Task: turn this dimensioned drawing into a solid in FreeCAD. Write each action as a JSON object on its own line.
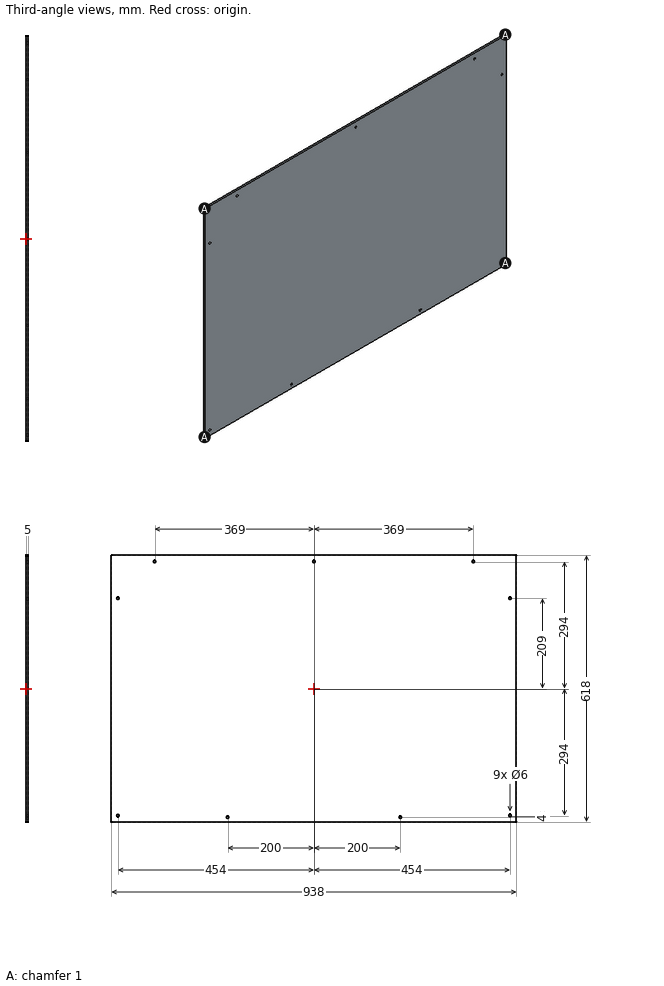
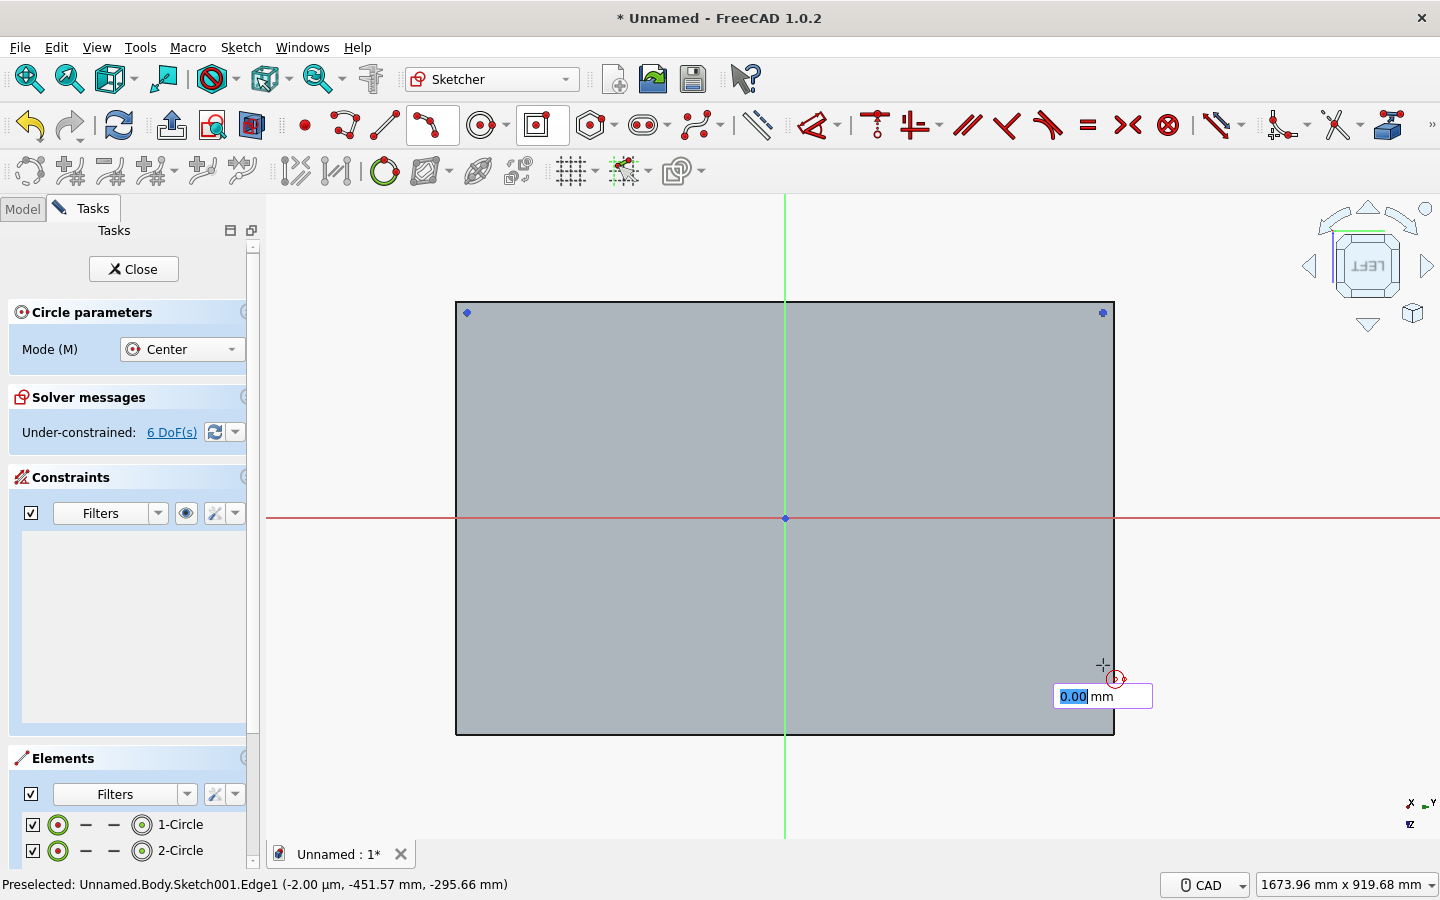
{"action": "scroll", "coordinate": [1105, 663], "scroll_direction": "up", "scroll_amount": 11}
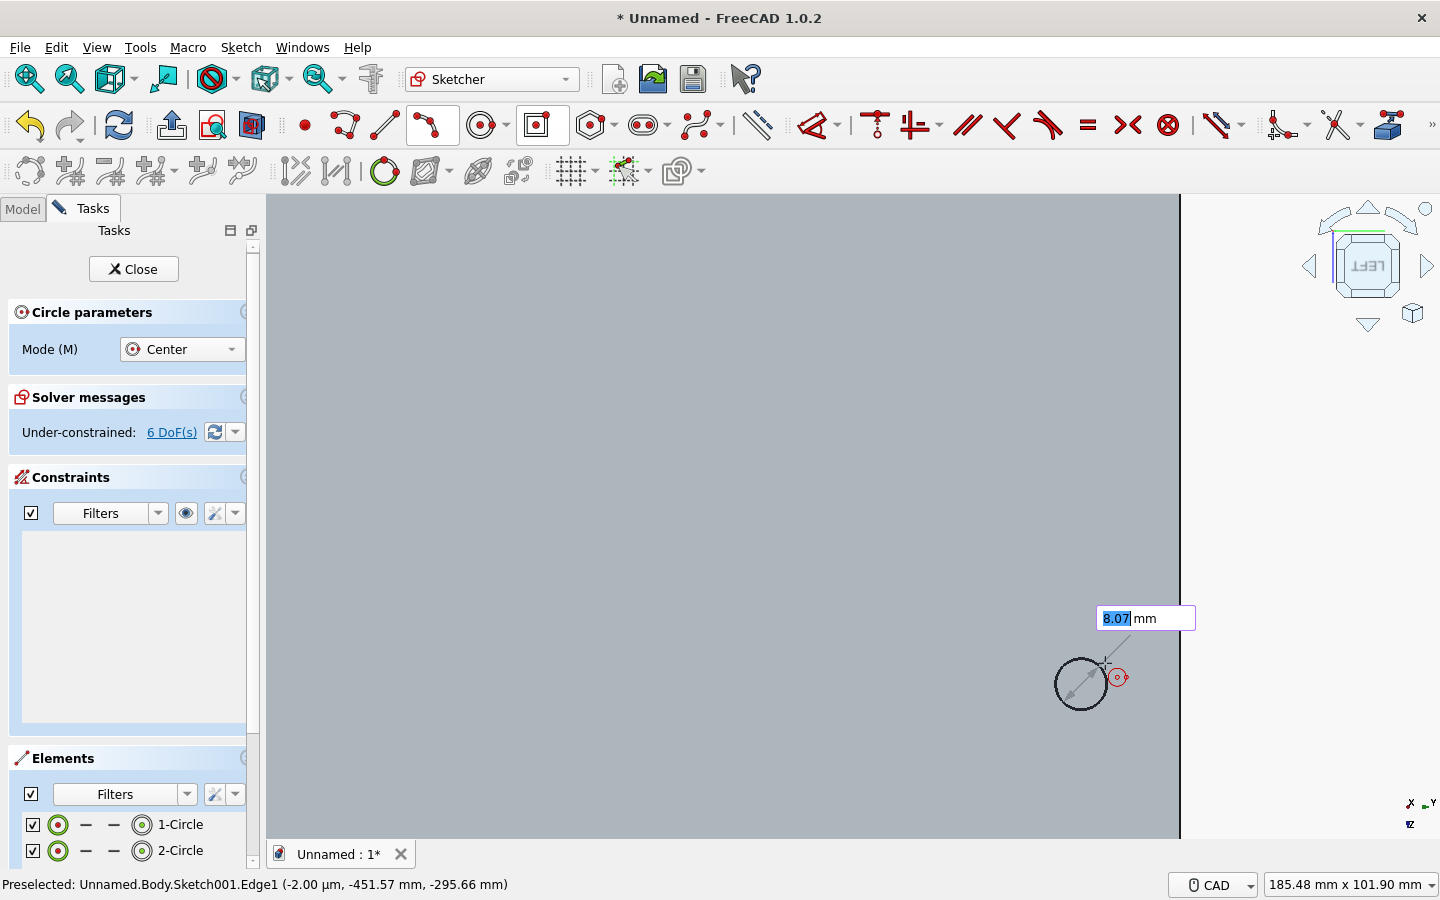
{"action": "left_click", "coordinate": [1099, 660]}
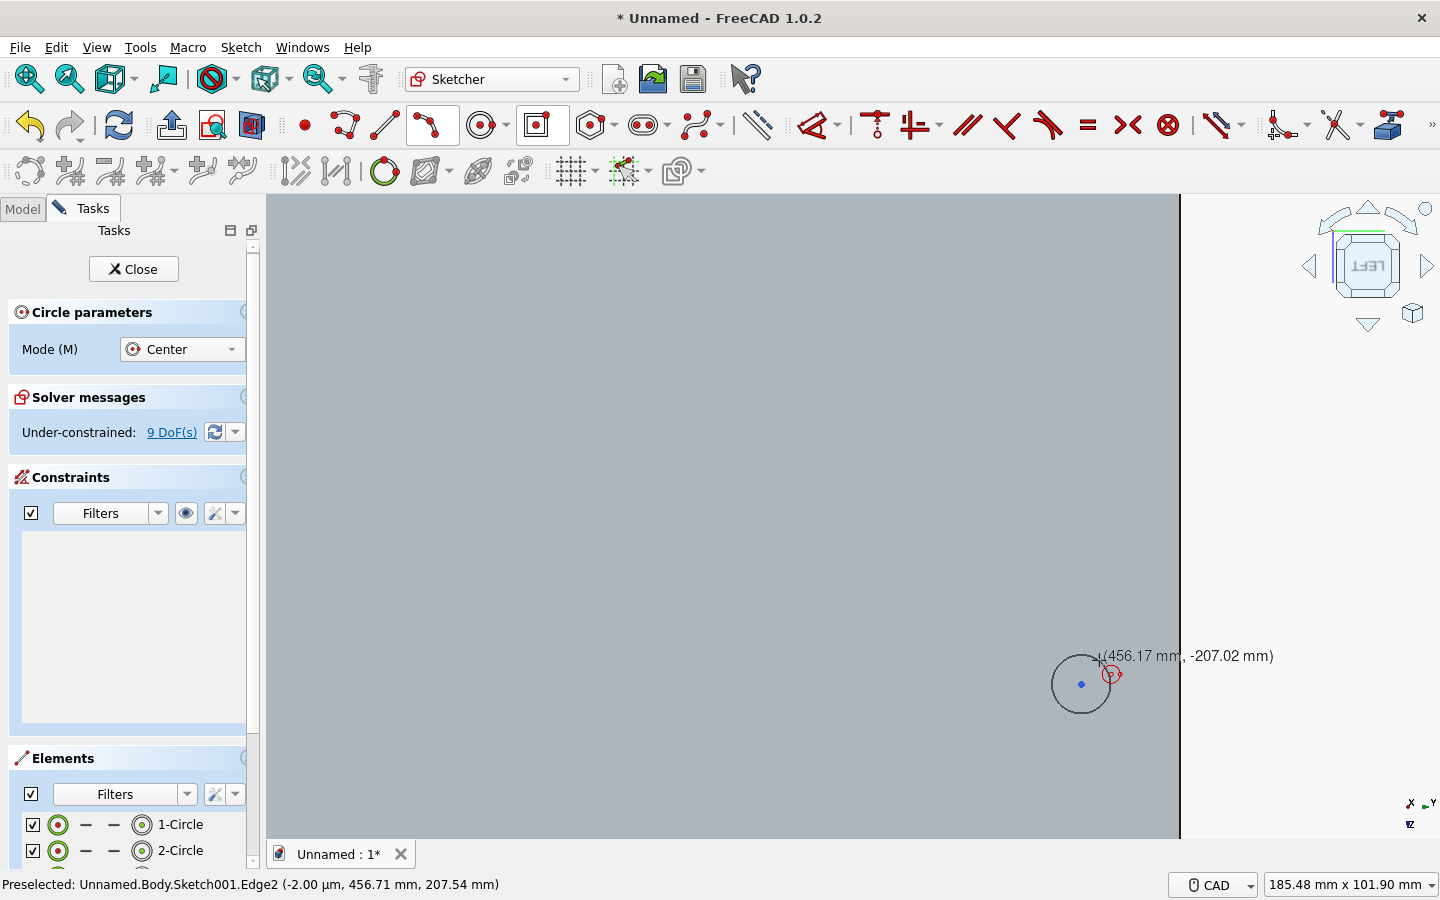
{"action": "scroll", "coordinate": [1105, 663], "scroll_direction": "down", "scroll_amount": 11}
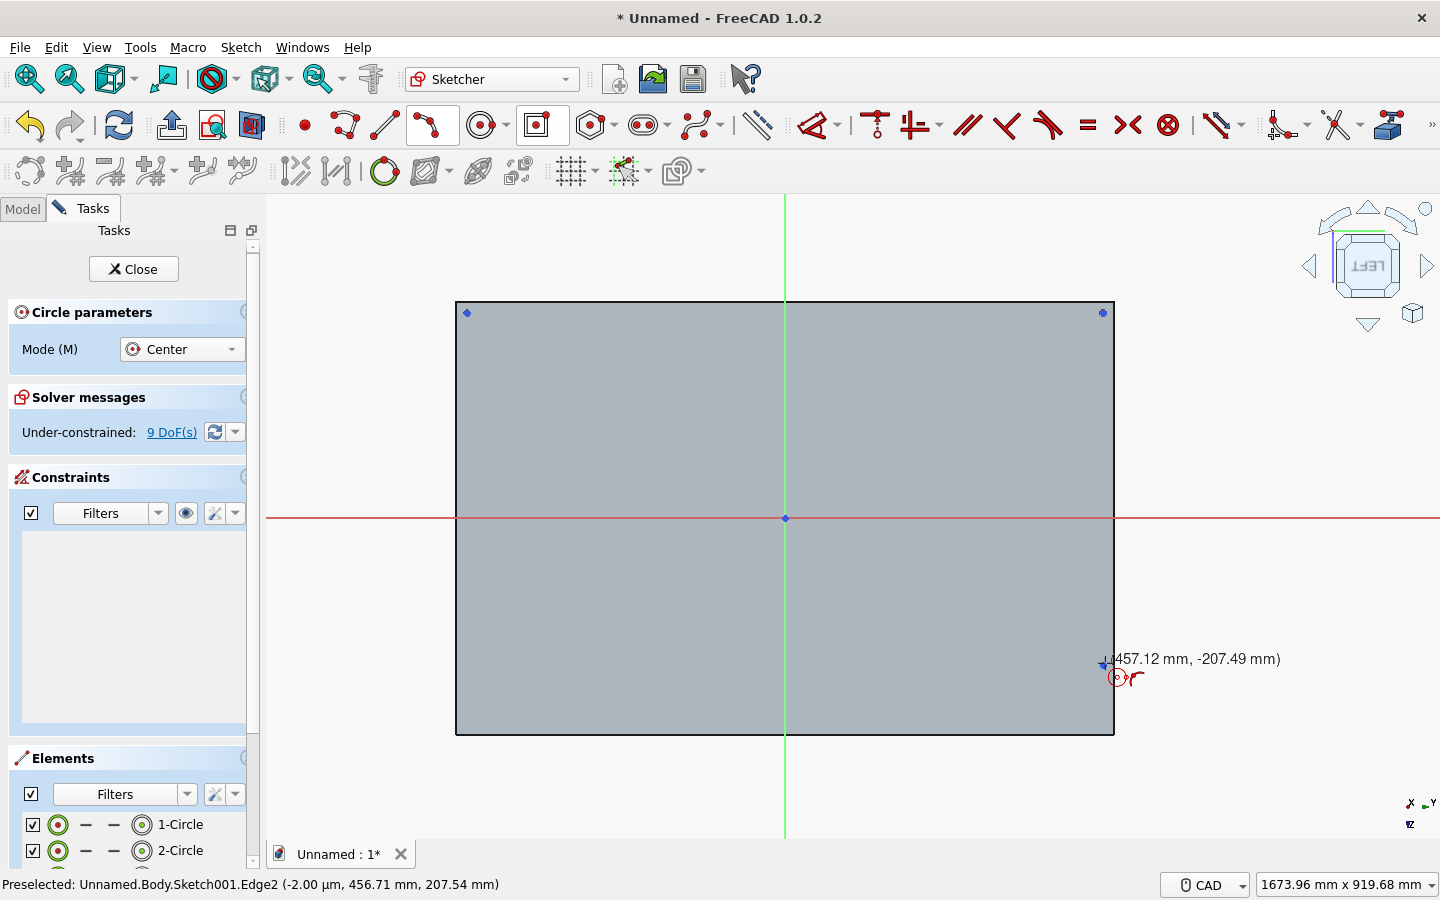
{"action": "scroll", "coordinate": [1044, 724], "scroll_direction": "up", "scroll_amount": 12}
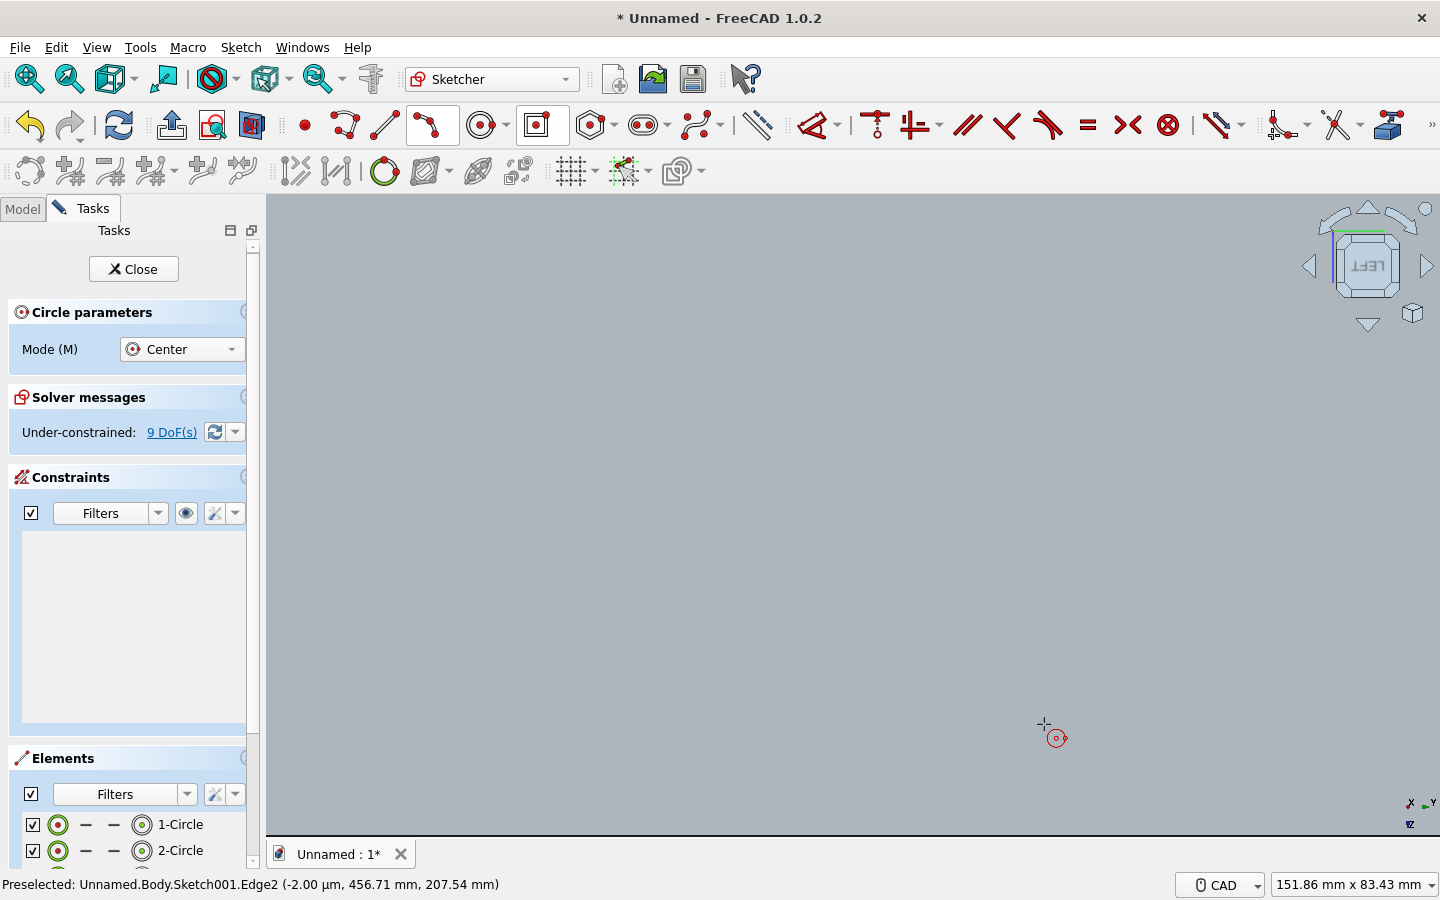
{"action": "scroll", "coordinate": [1044, 724], "scroll_direction": "down", "scroll_amount": 12}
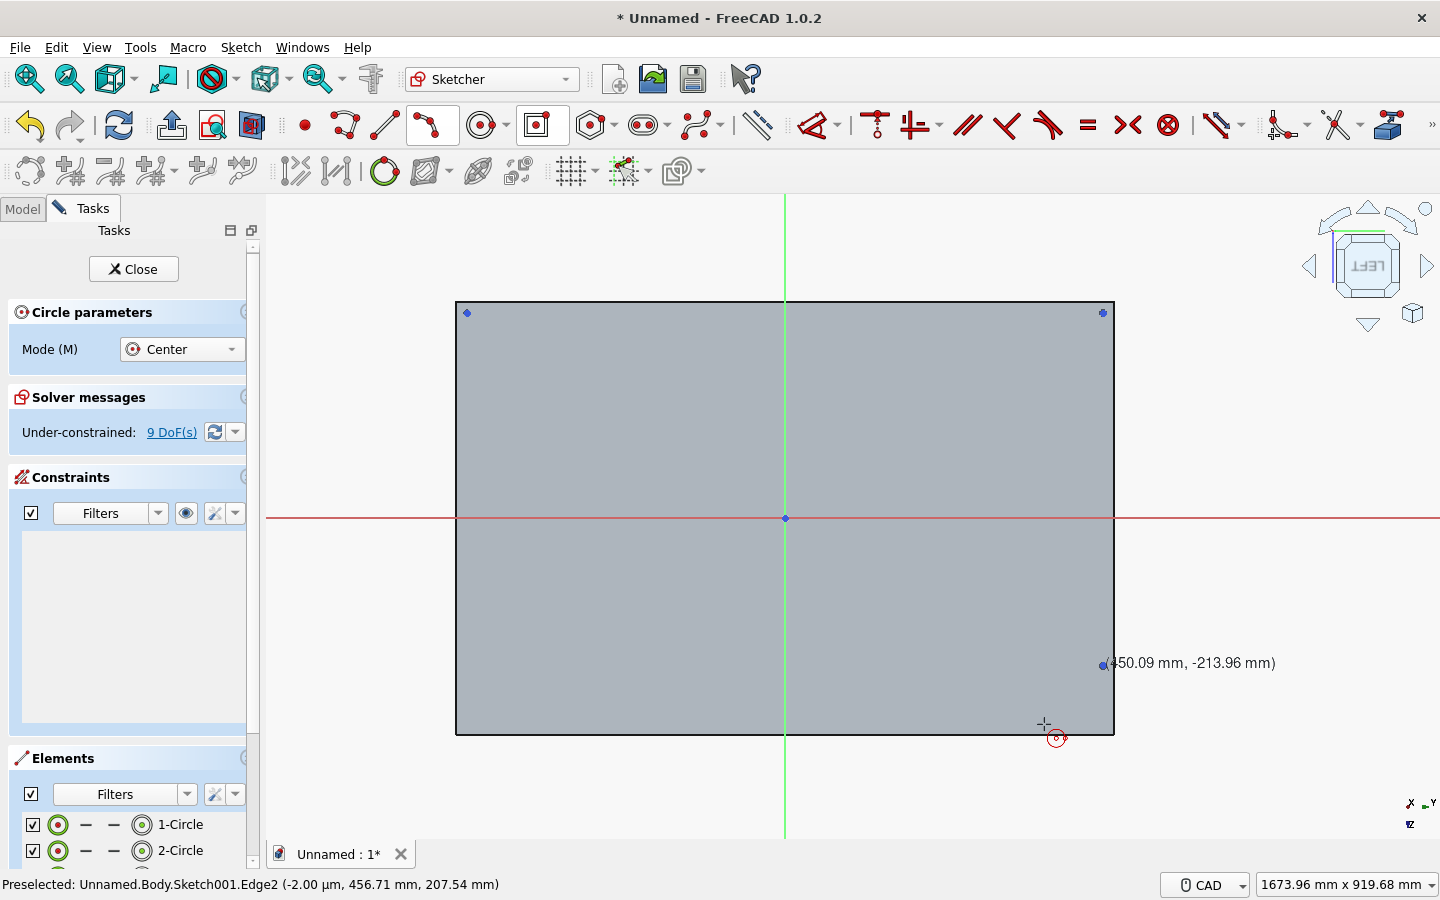
{"action": "left_click", "coordinate": [1044, 724]}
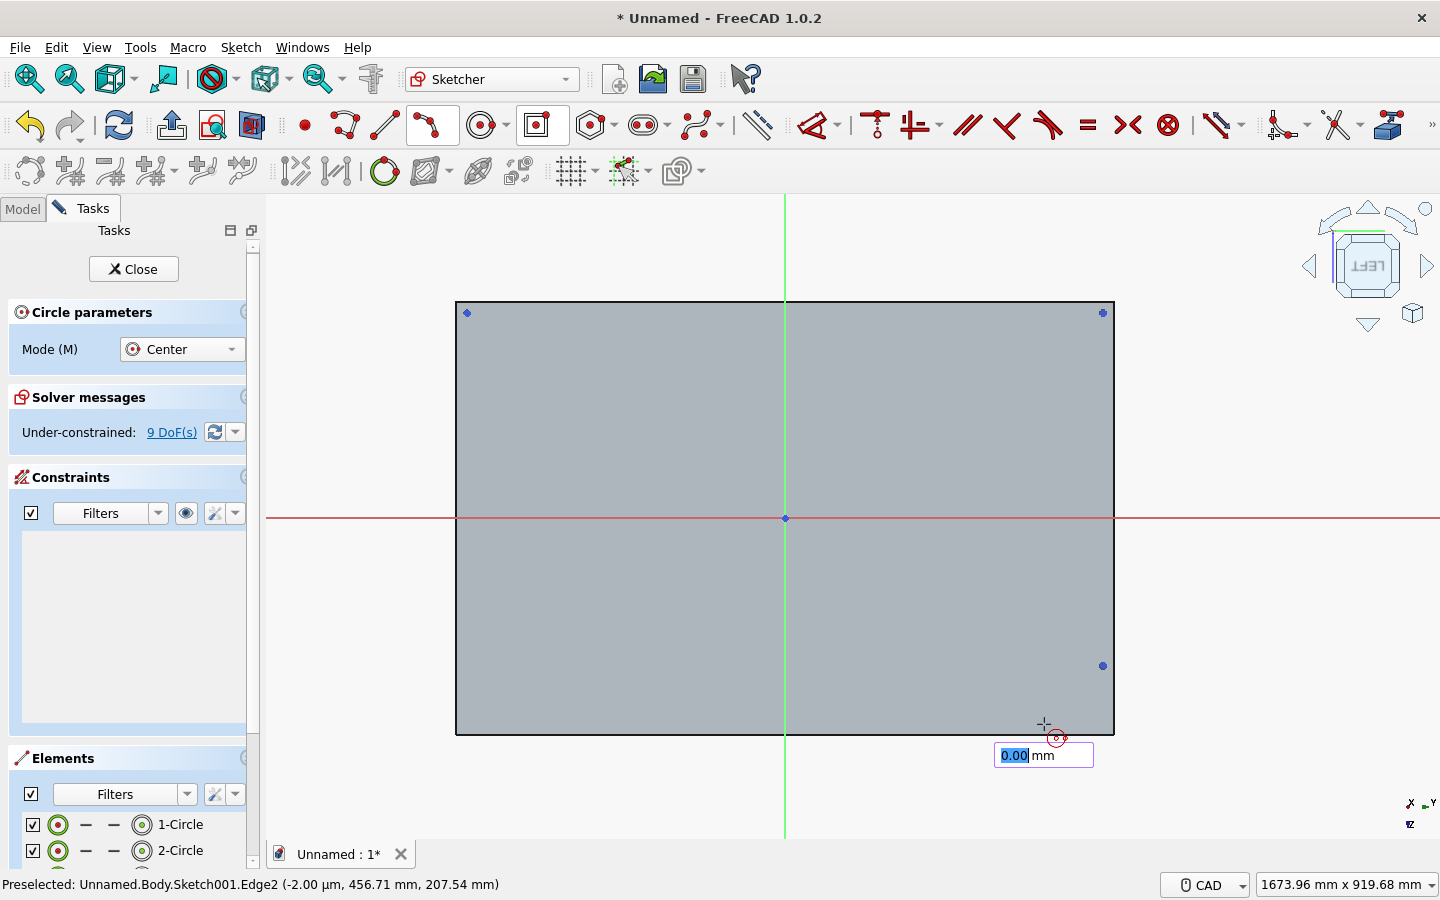
{"action": "scroll", "coordinate": [1045, 723], "scroll_direction": "up", "scroll_amount": 11}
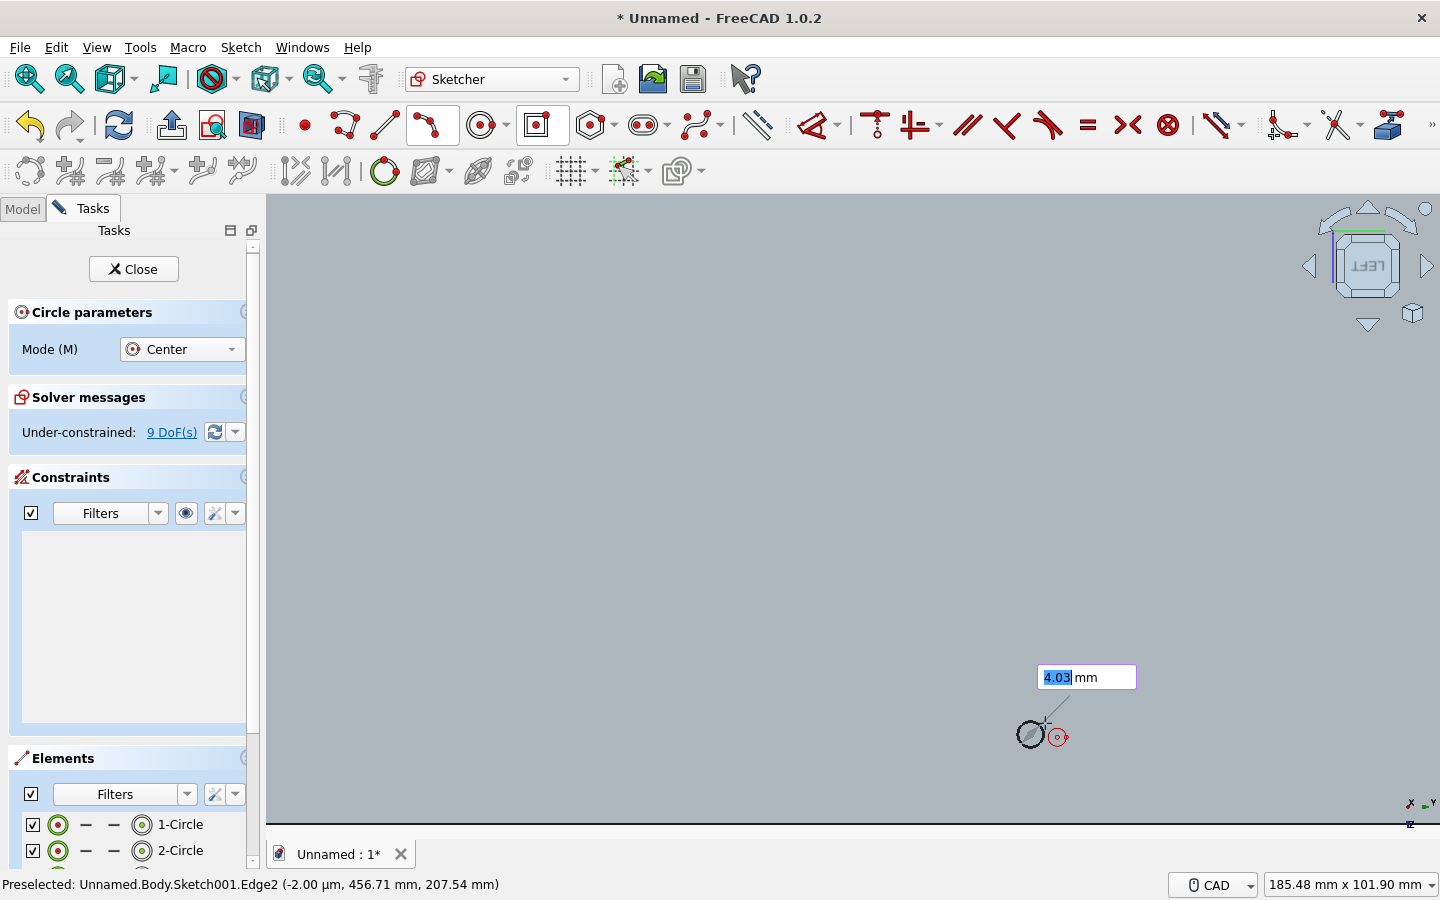
{"action": "left_click", "coordinate": [1043, 716]}